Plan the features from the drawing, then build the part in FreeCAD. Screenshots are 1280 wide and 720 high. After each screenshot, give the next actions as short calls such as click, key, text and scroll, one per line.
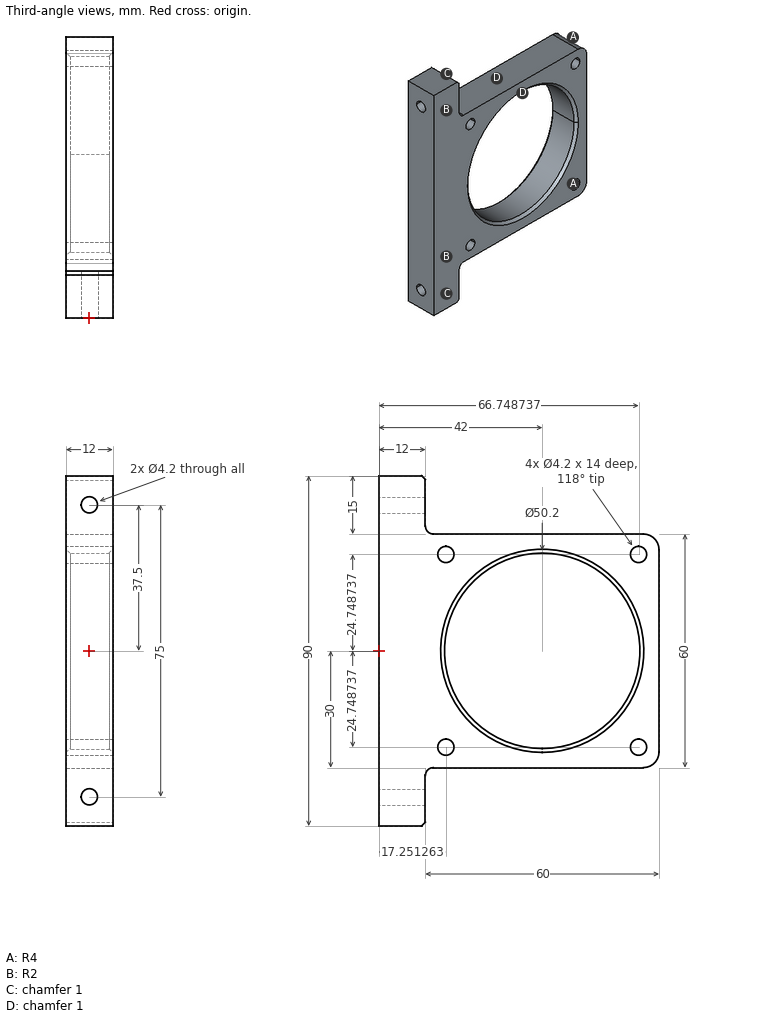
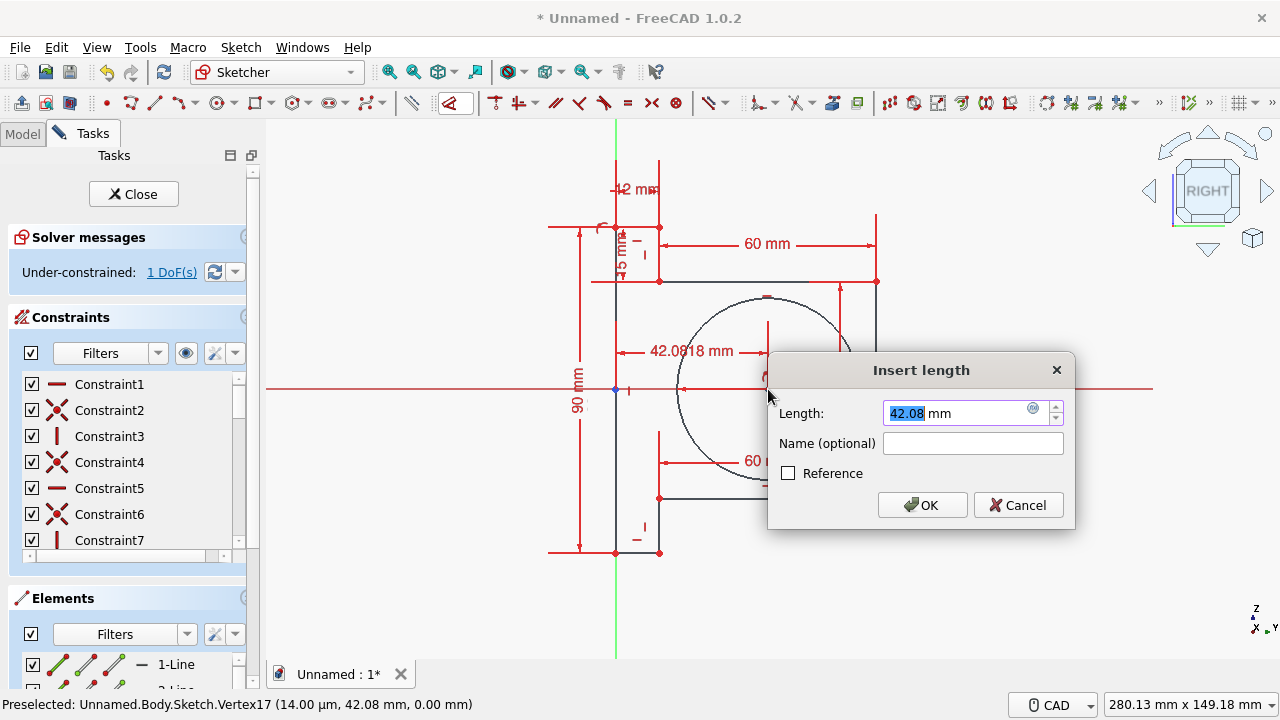
text(42)
key(Return)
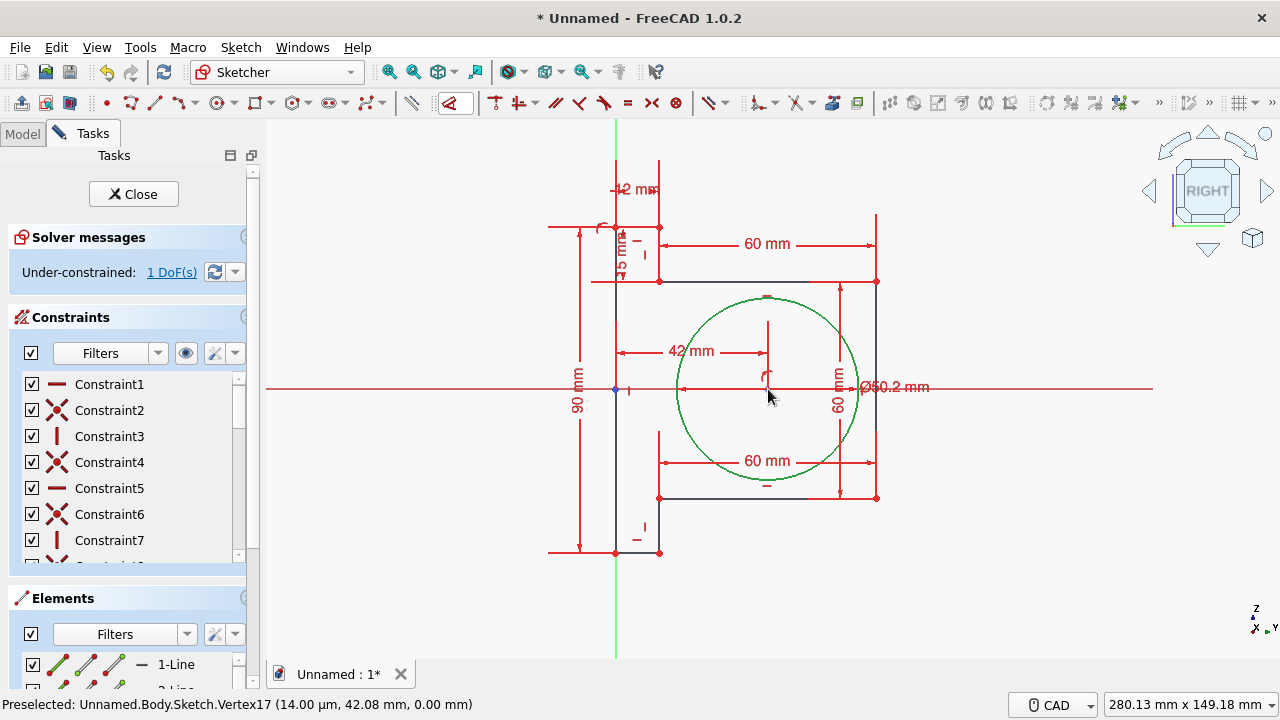
click(659, 499)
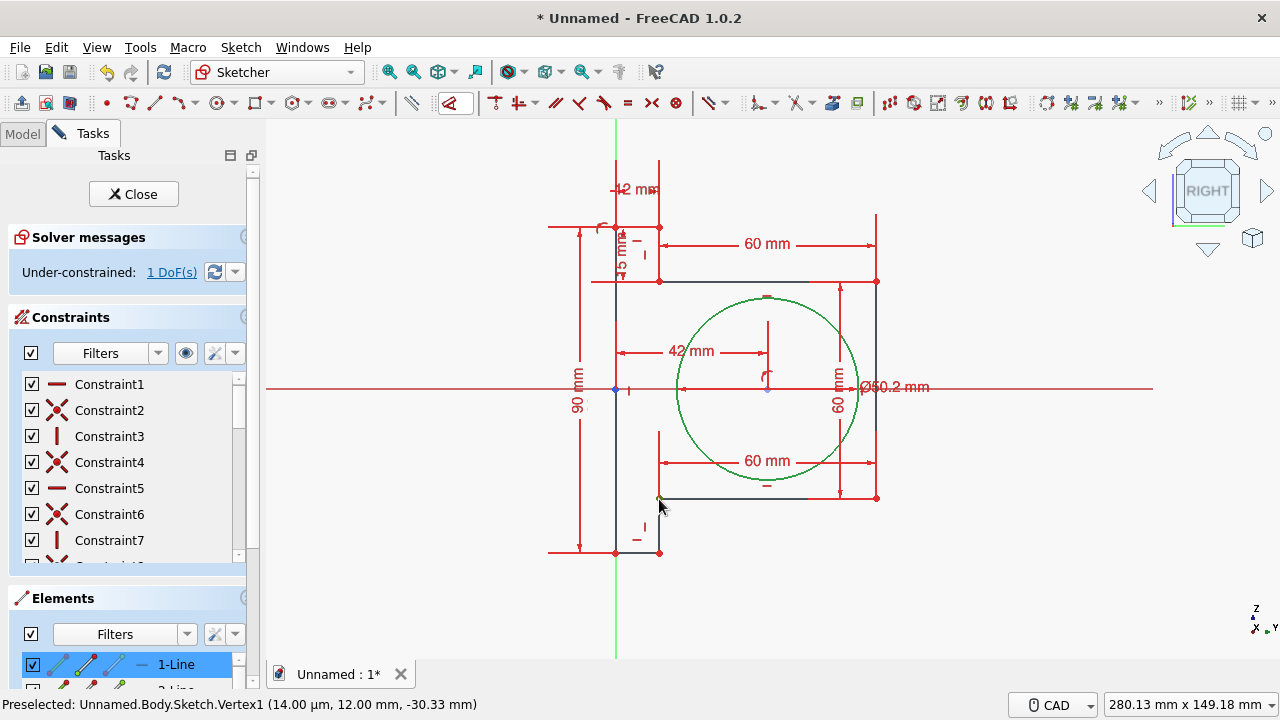
click(468, 104)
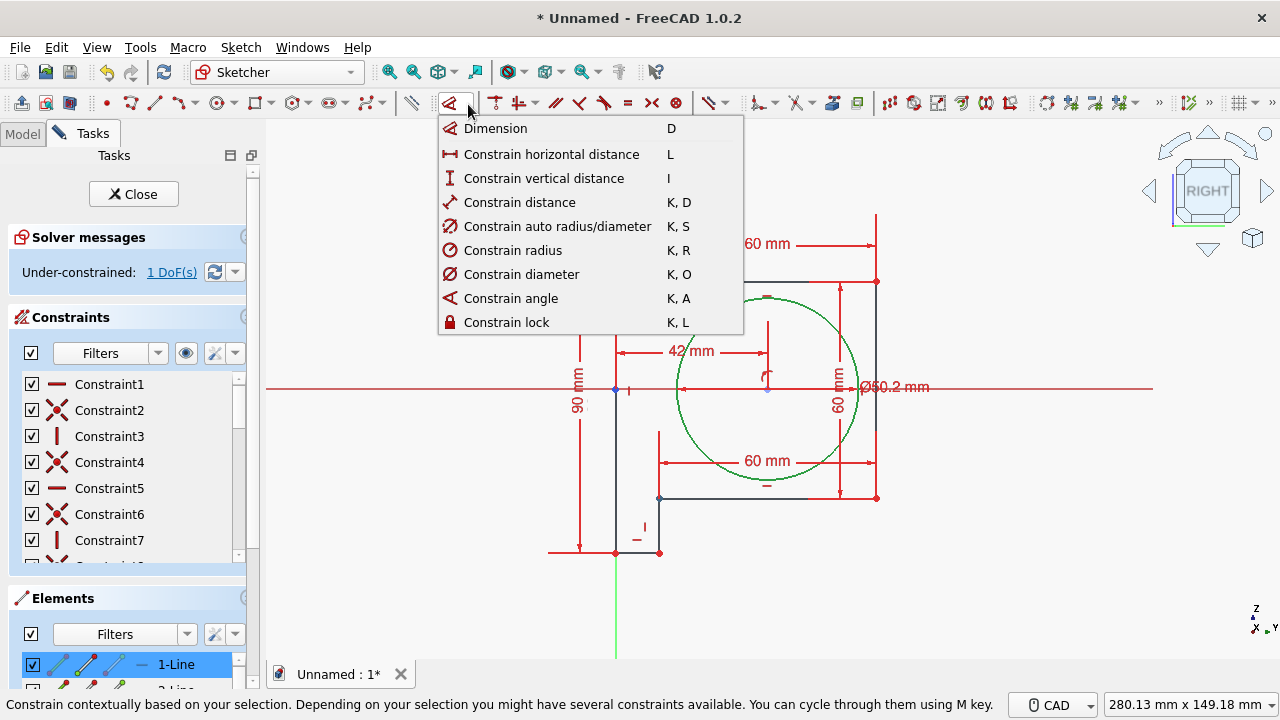
click(591, 178)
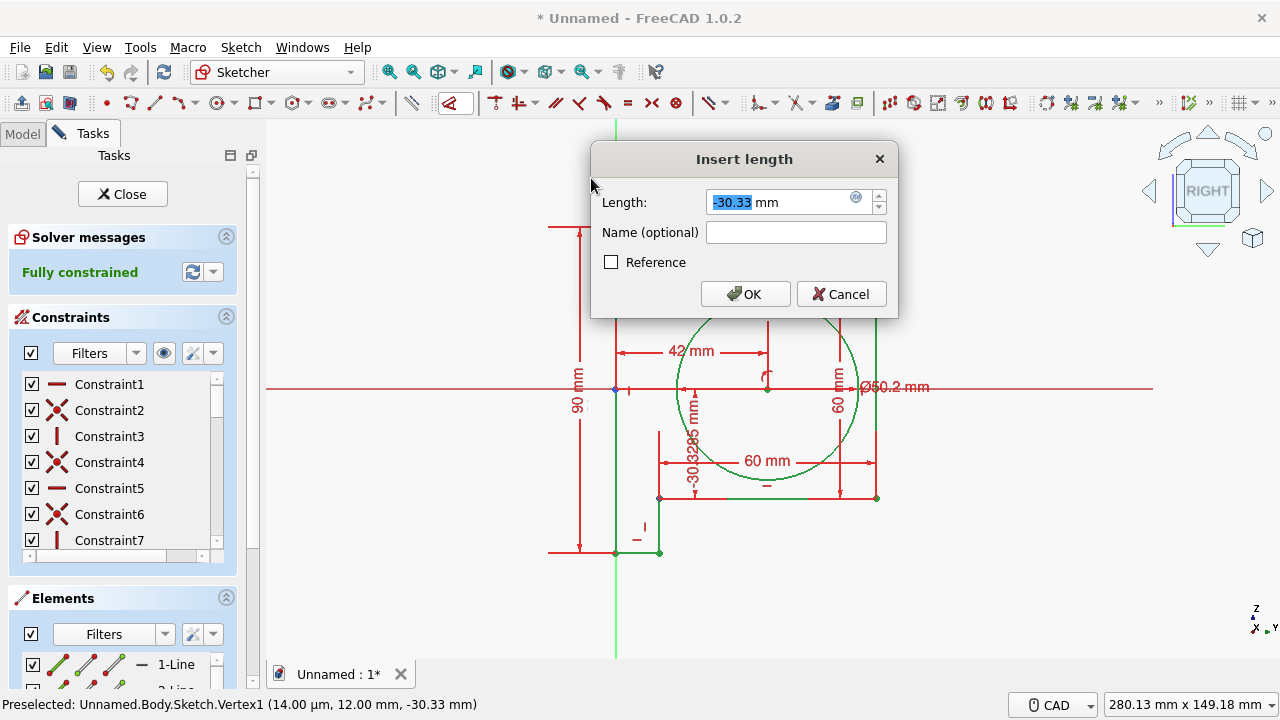
text(-30)
key(Return)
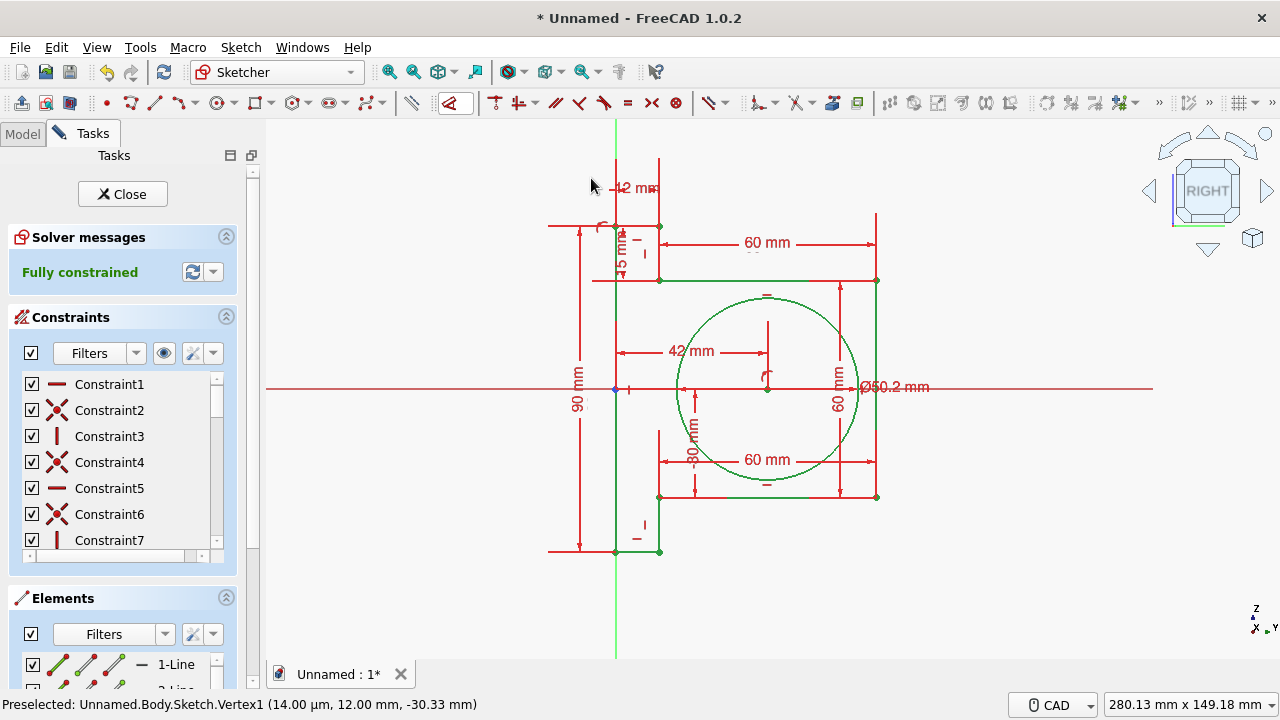
click(123, 194)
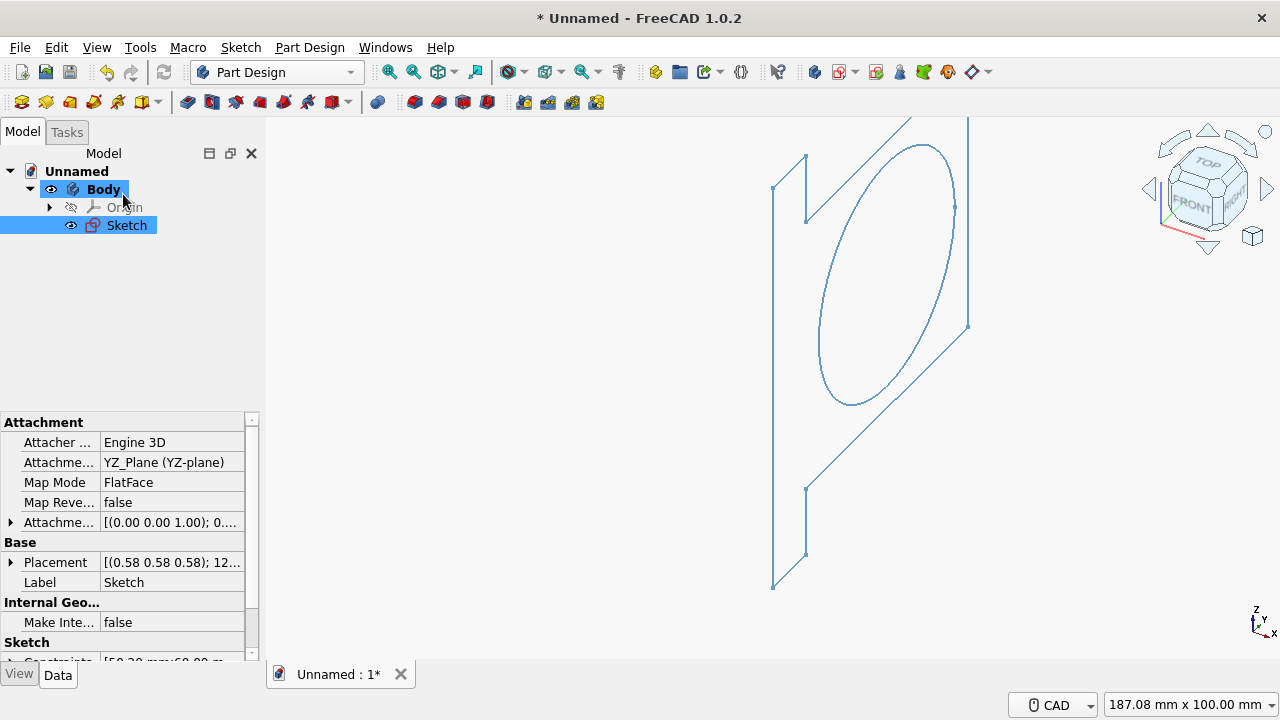
click(22, 102)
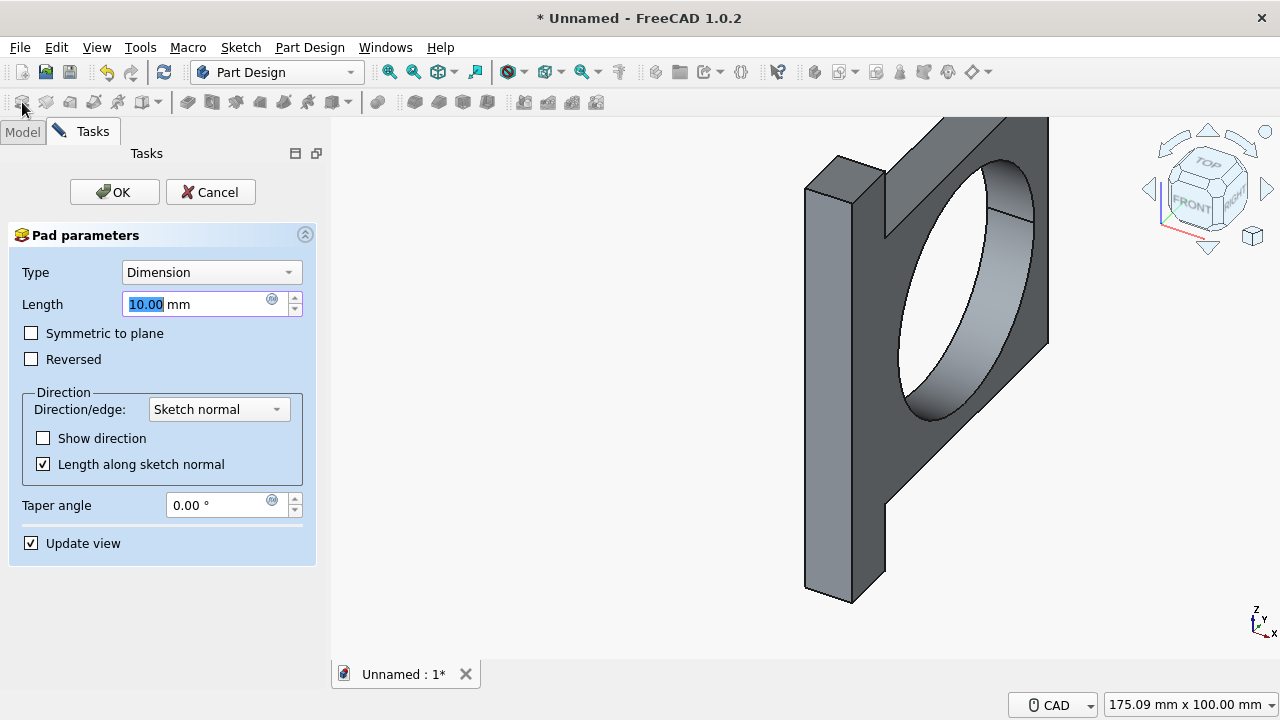
text(12)
key(Tab)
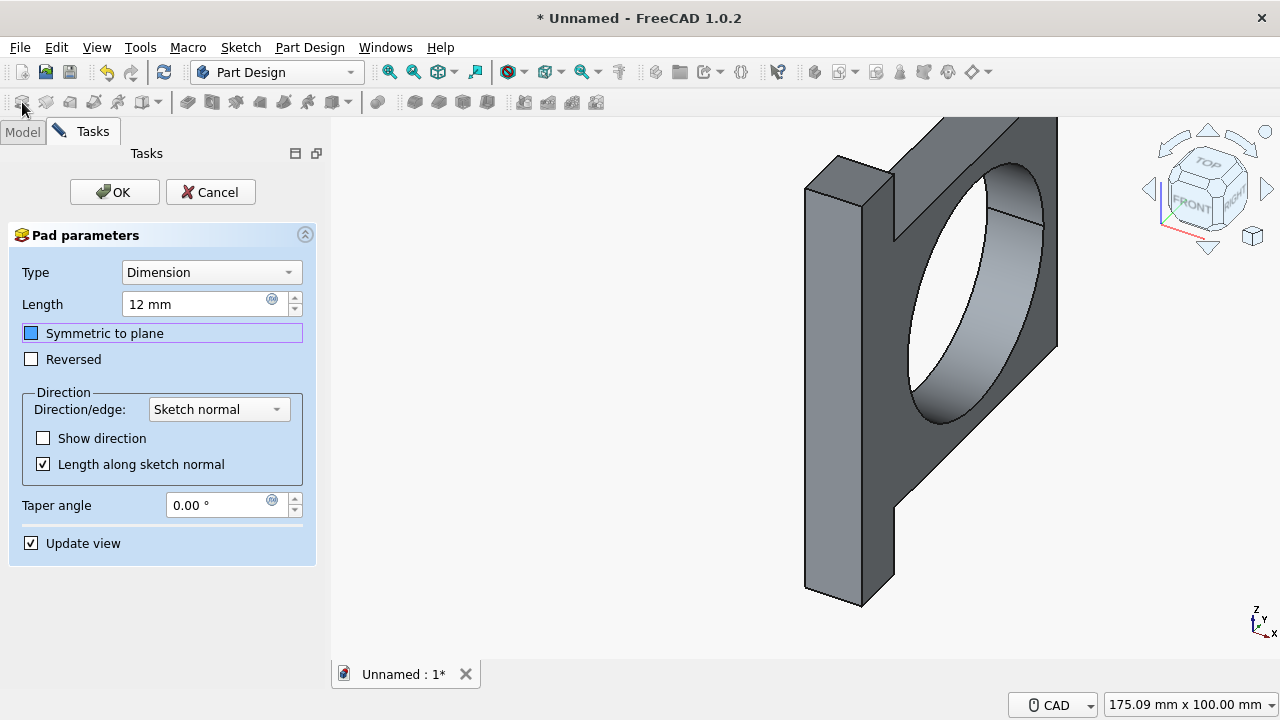
click(30, 333)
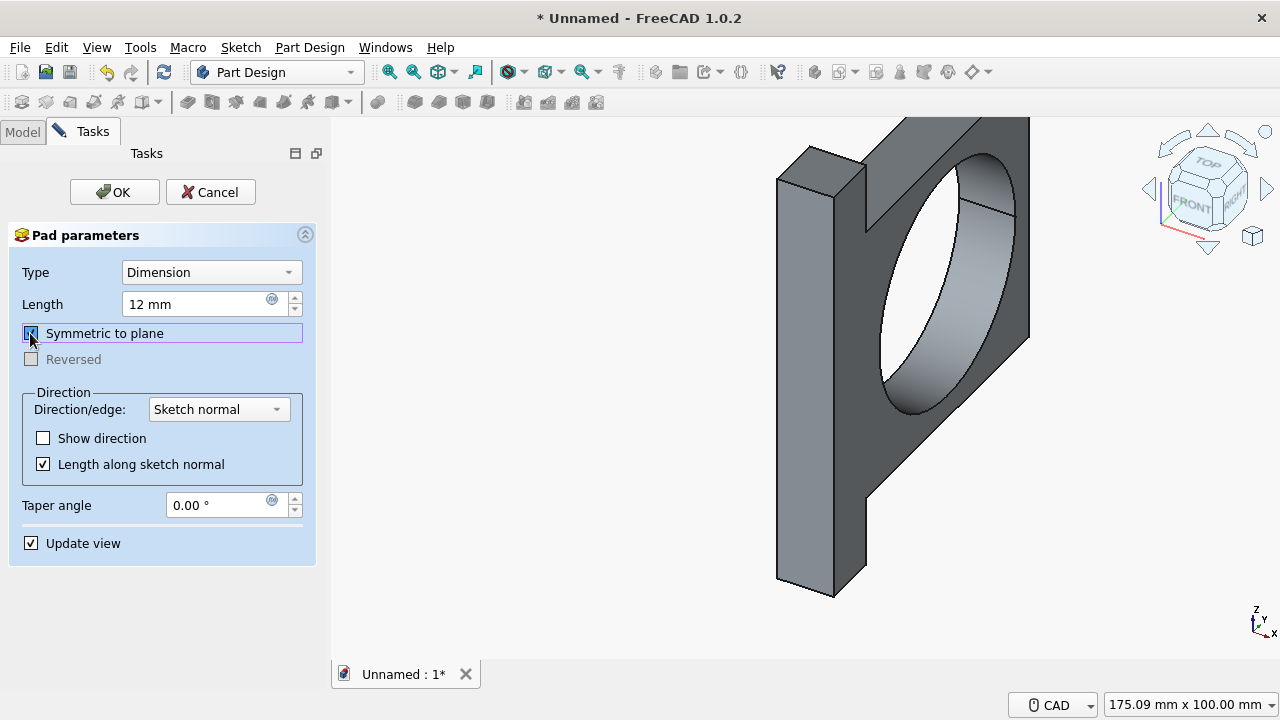
click(115, 192)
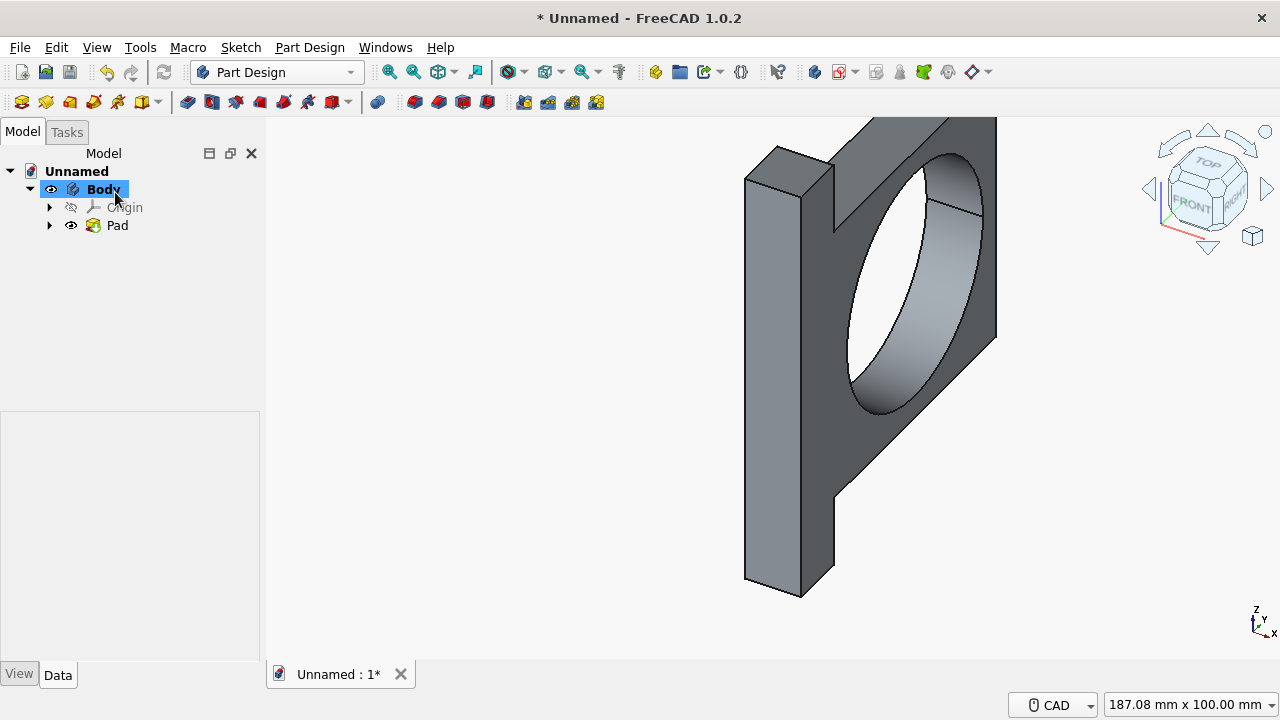
click(390, 72)